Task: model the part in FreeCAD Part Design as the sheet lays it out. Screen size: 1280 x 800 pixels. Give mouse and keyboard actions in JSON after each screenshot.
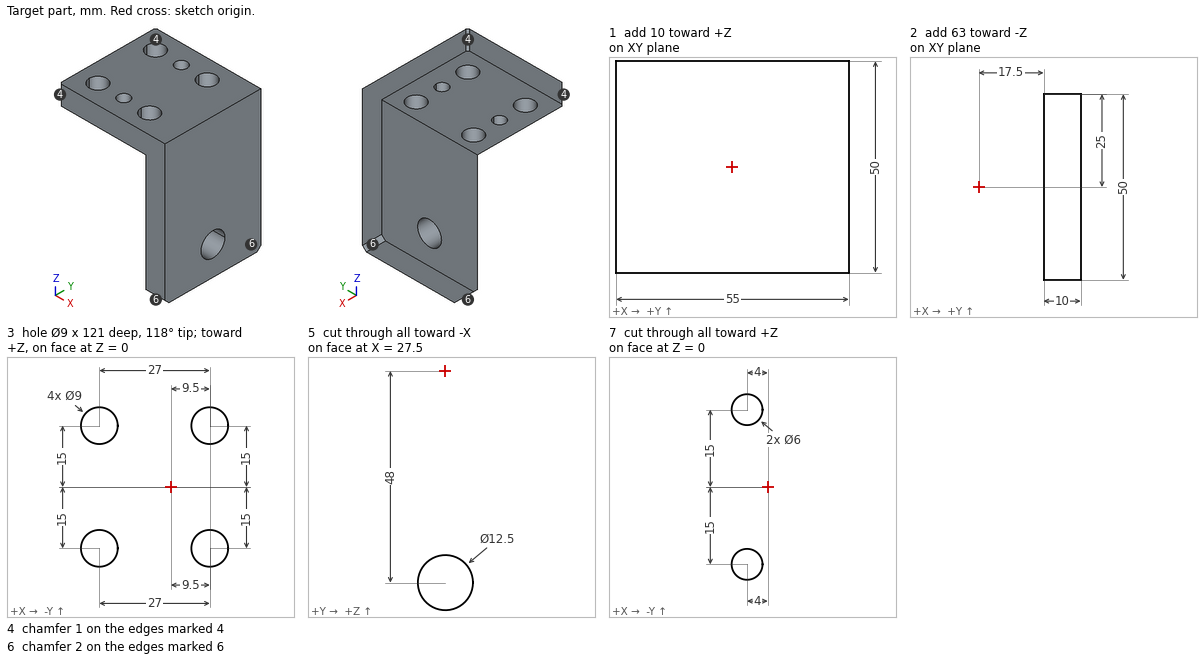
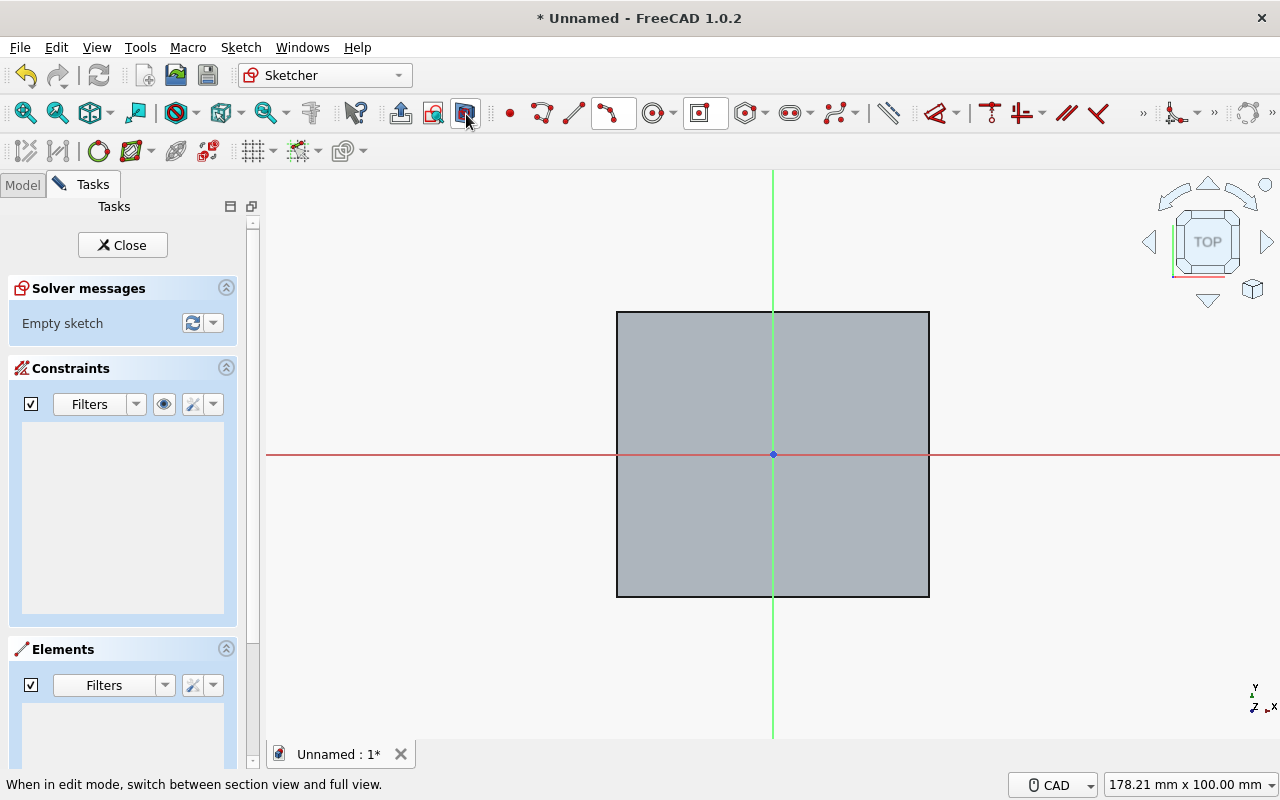
{"action": "key", "text": "g r"}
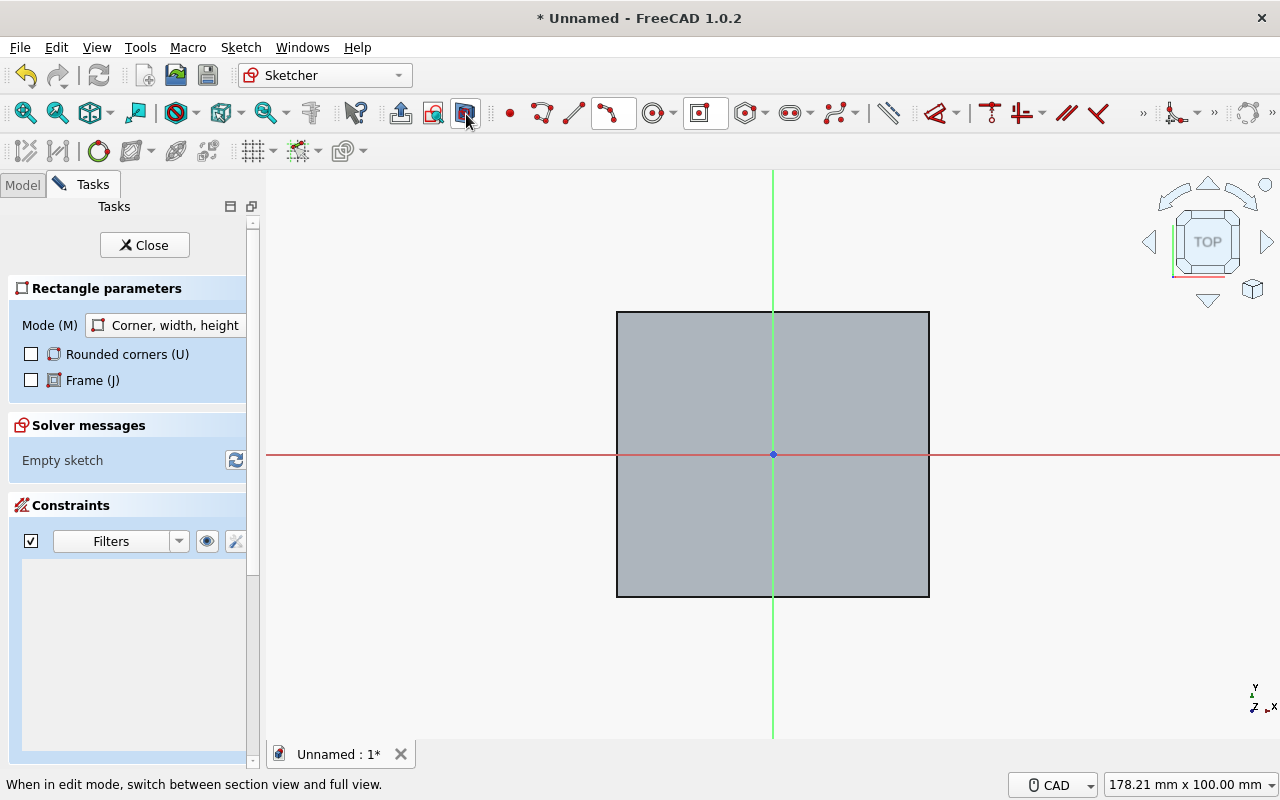
{"action": "left_click", "coordinate": [873, 312]}
{"action": "left_click", "coordinate": [929, 597]}
{"action": "key", "text": "Escape"}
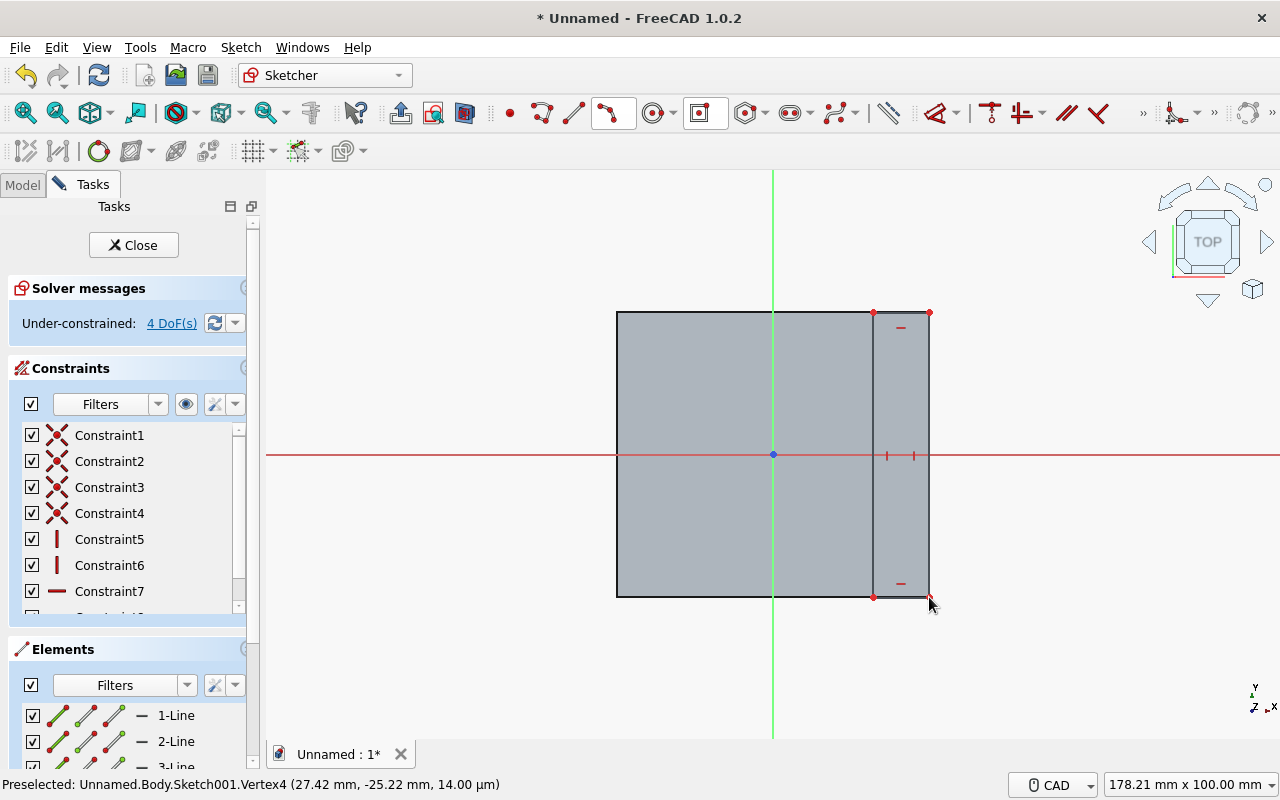
{"action": "left_click", "coordinate": [936, 114]}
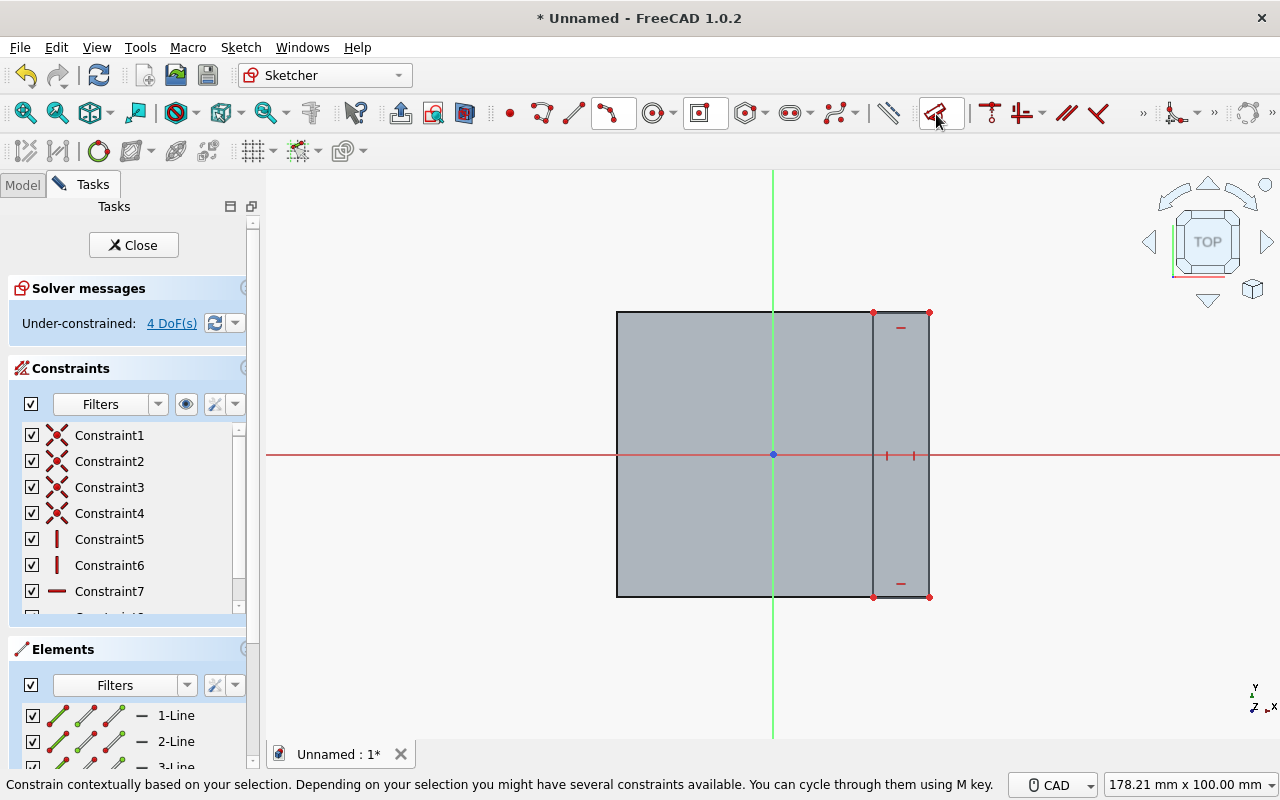
{"action": "left_click", "coordinate": [873, 398]}
{"action": "left_click", "coordinate": [907, 390]}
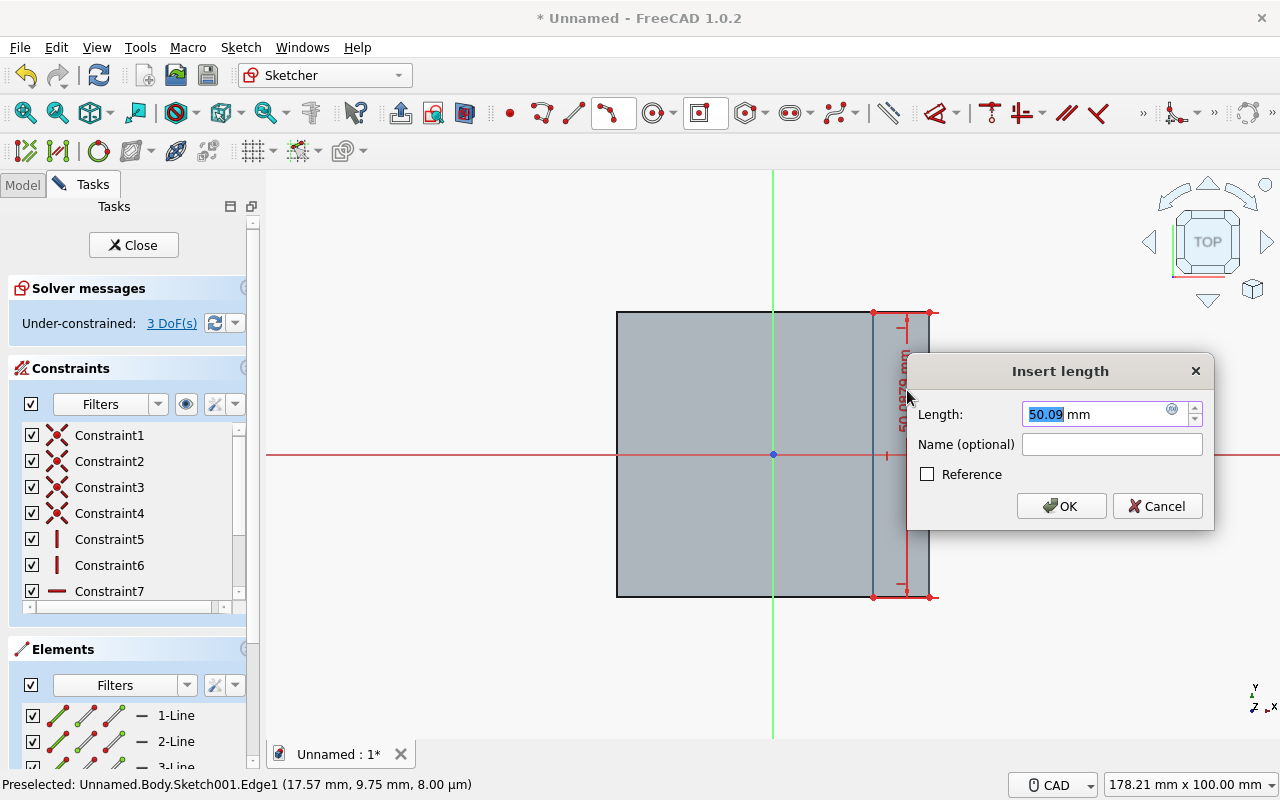
{"action": "type", "text": "50"}
{"action": "key", "text": "Return"}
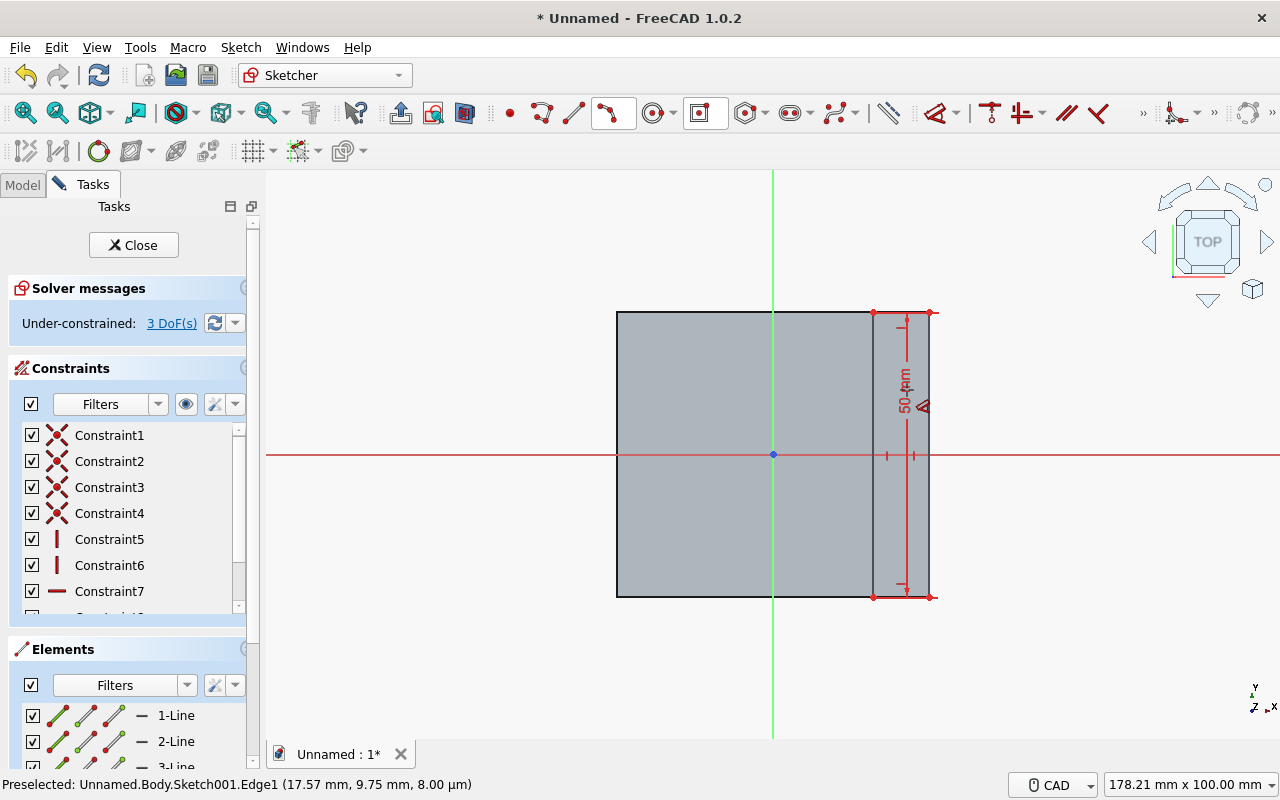
{"action": "left_click", "coordinate": [890, 597]}
{"action": "left_click", "coordinate": [901, 631]}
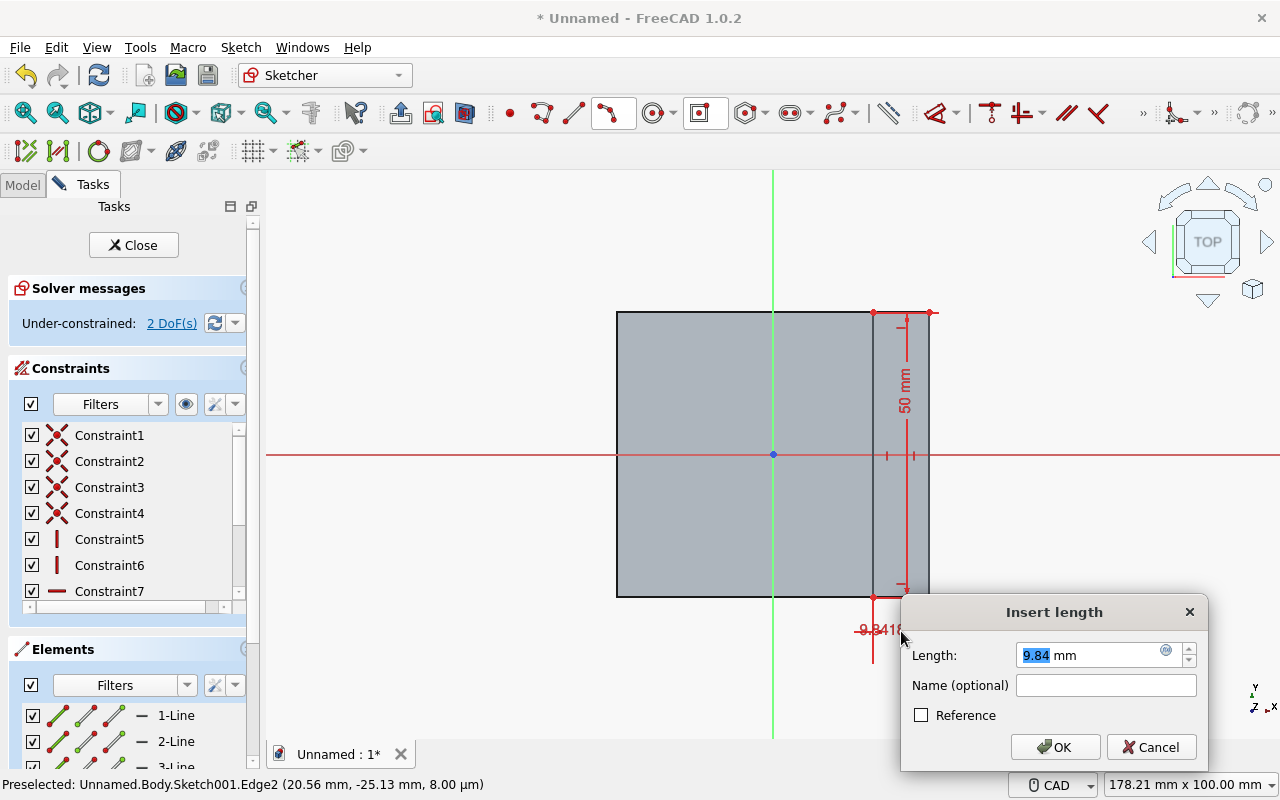
{"action": "type", "text": "10"}
{"action": "key", "text": "Return"}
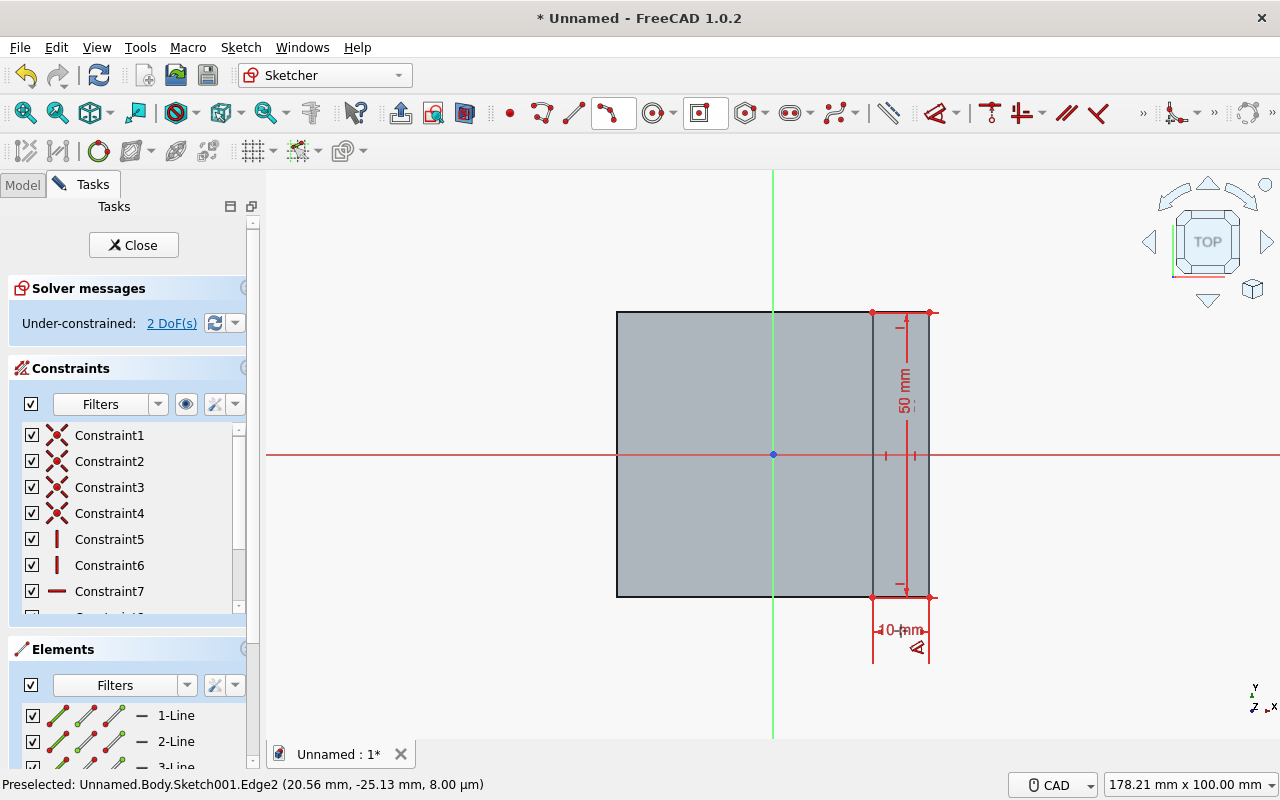
{"action": "left_click", "coordinate": [873, 313]}
{"action": "left_click", "coordinate": [739, 384]}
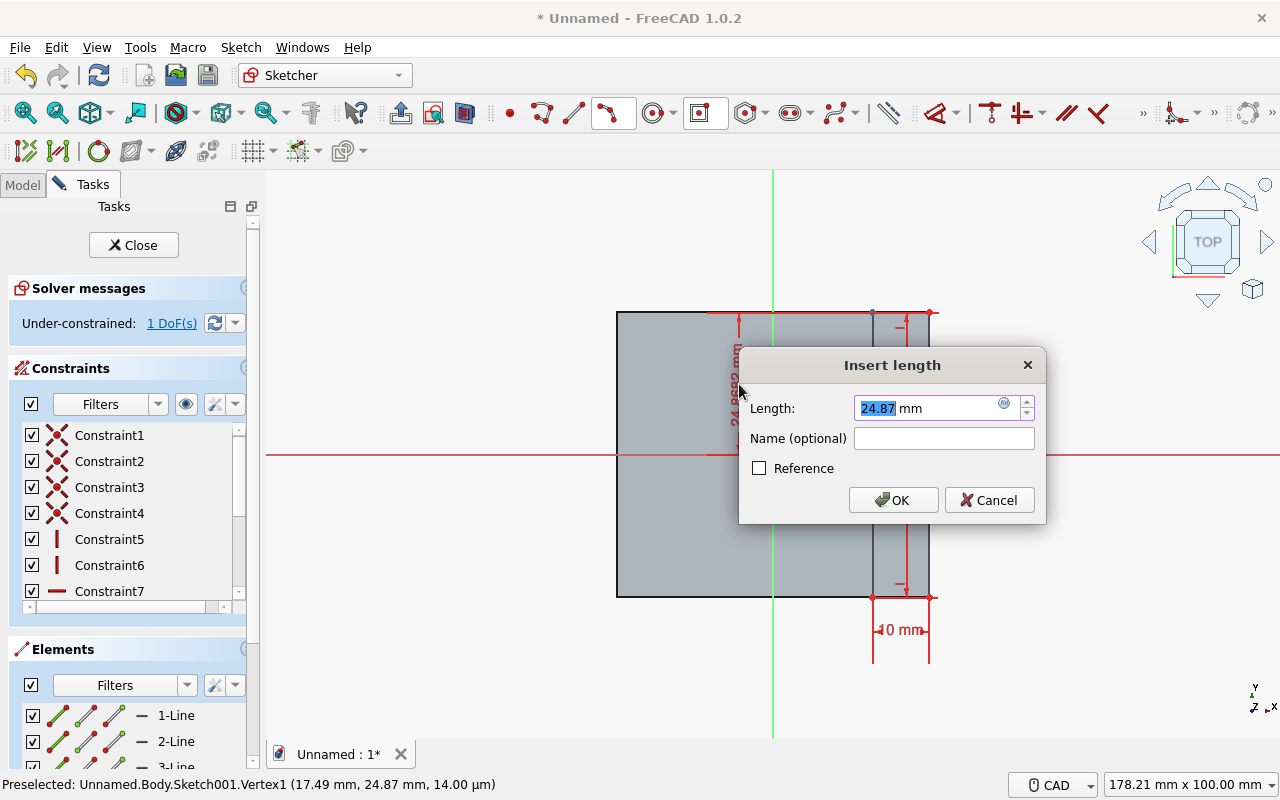
{"action": "type", "text": "25"}
{"action": "key", "text": "Return"}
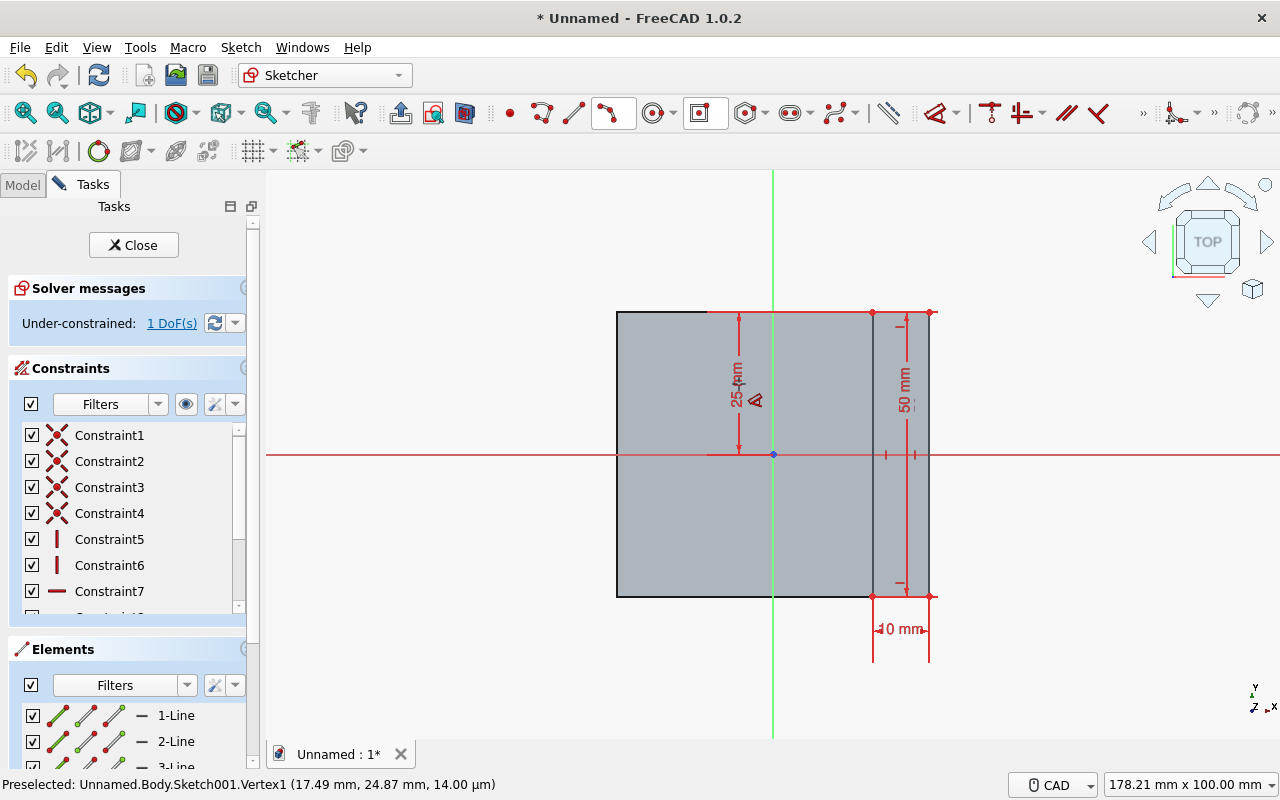
{"action": "left_click", "coordinate": [873, 312]}
{"action": "left_click", "coordinate": [823, 278]}